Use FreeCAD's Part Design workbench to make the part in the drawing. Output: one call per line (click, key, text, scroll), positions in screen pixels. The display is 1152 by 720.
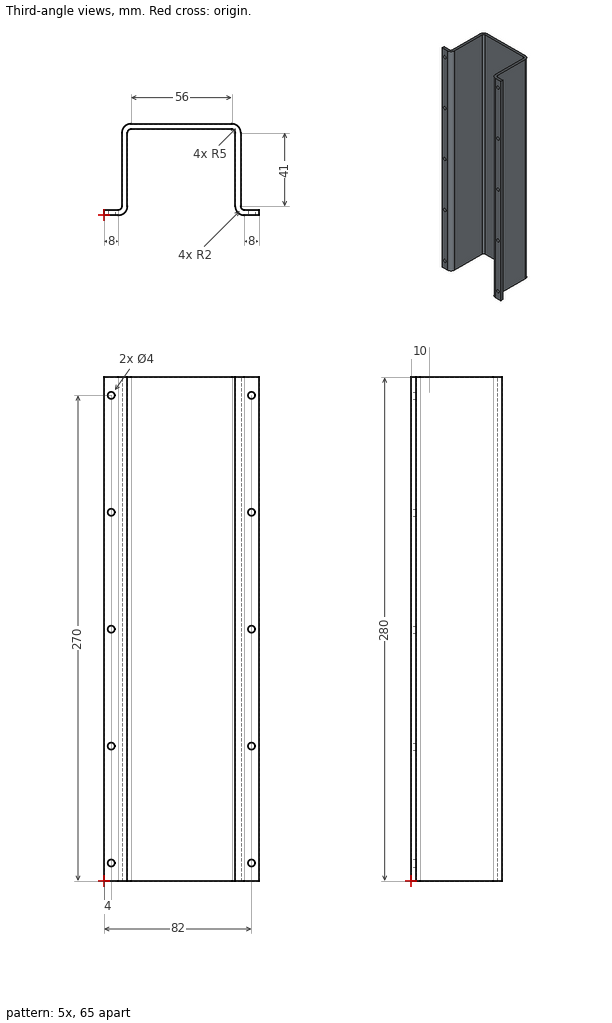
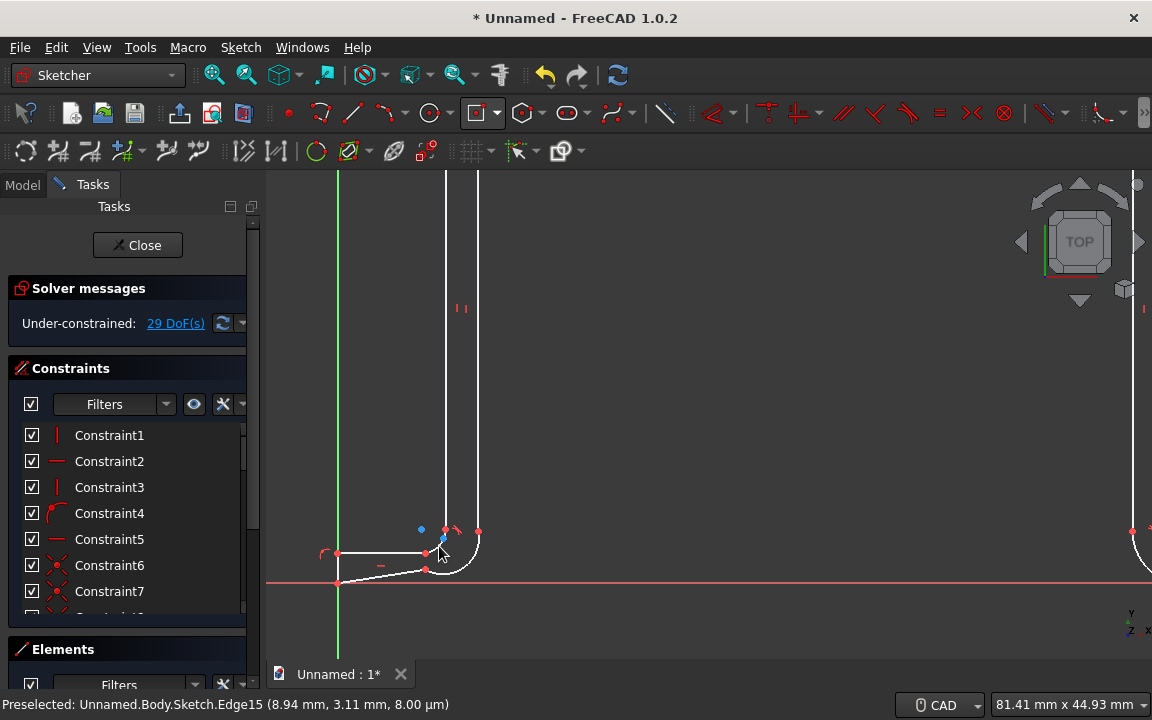
click(399, 553)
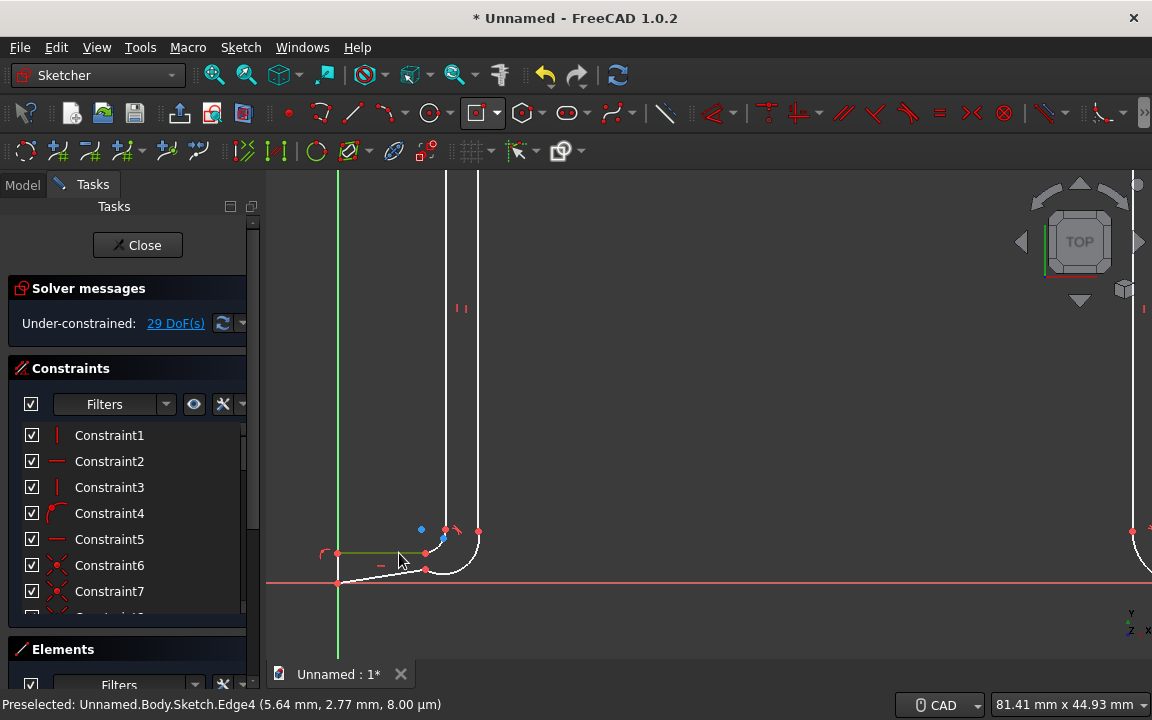
scroll(435, 550, up, 2)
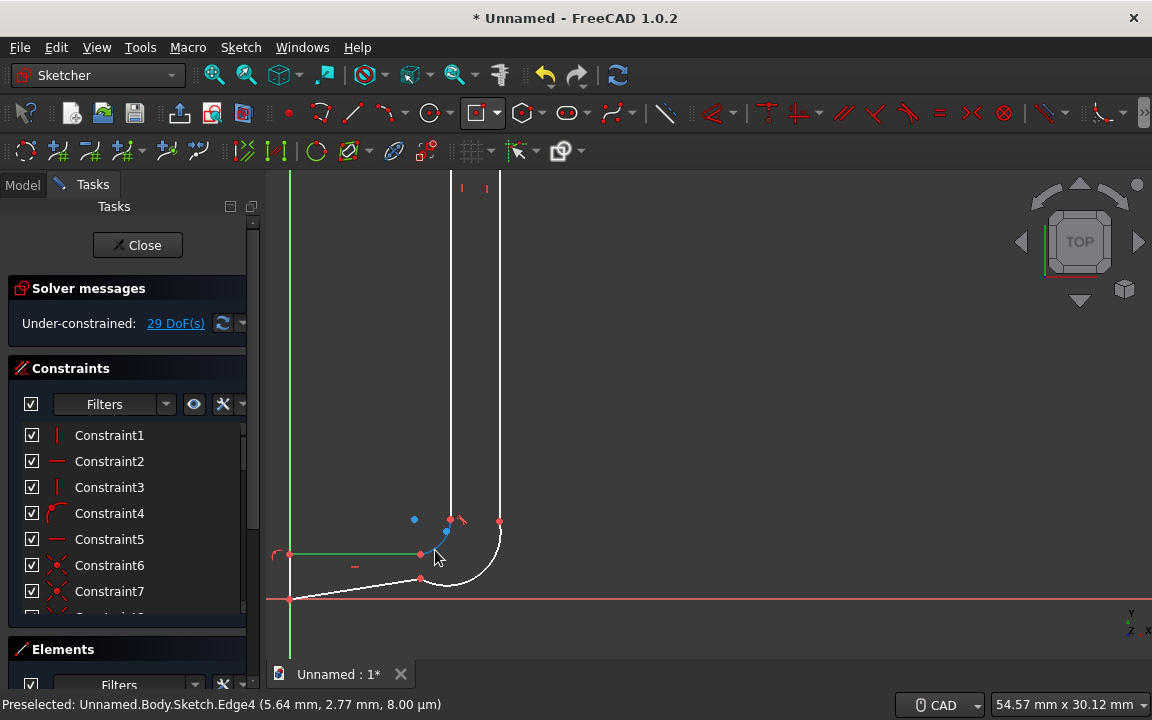
click(435, 549)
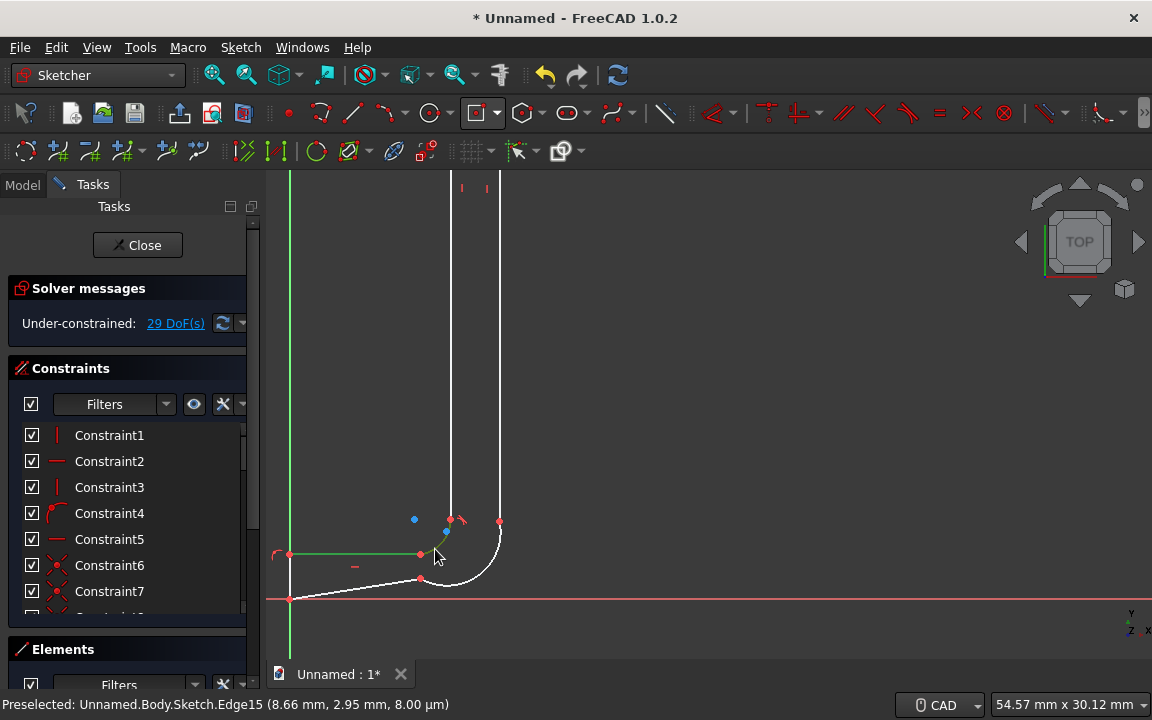
key(t)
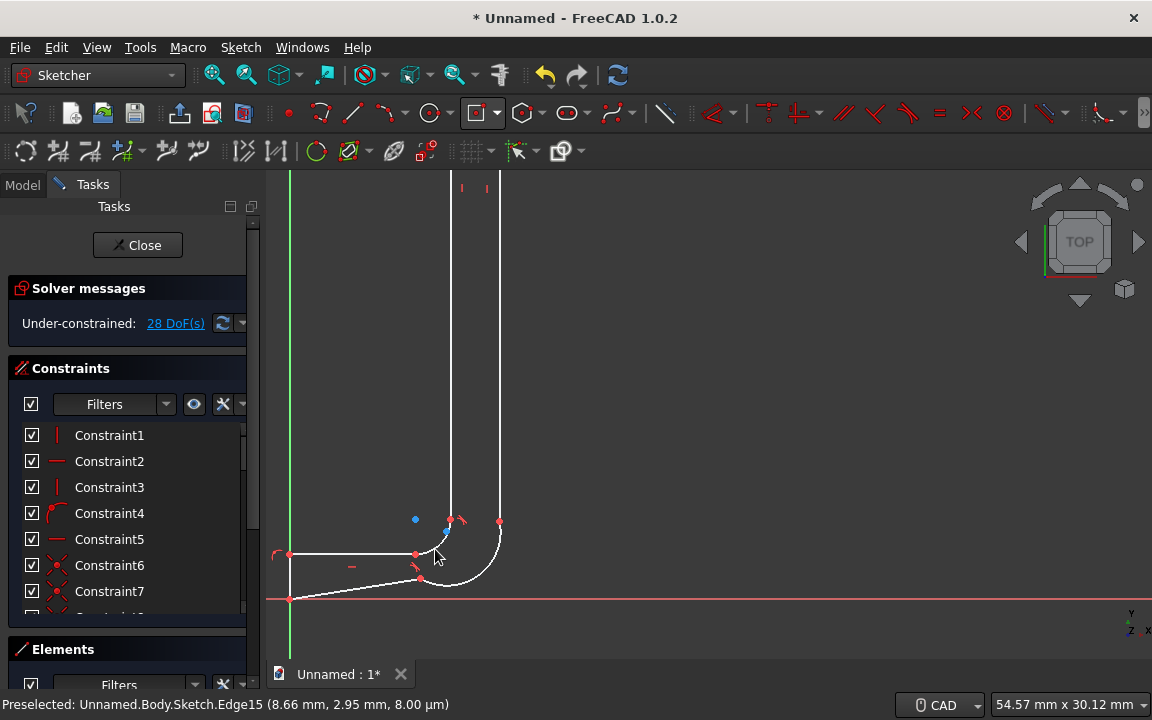
click(381, 585)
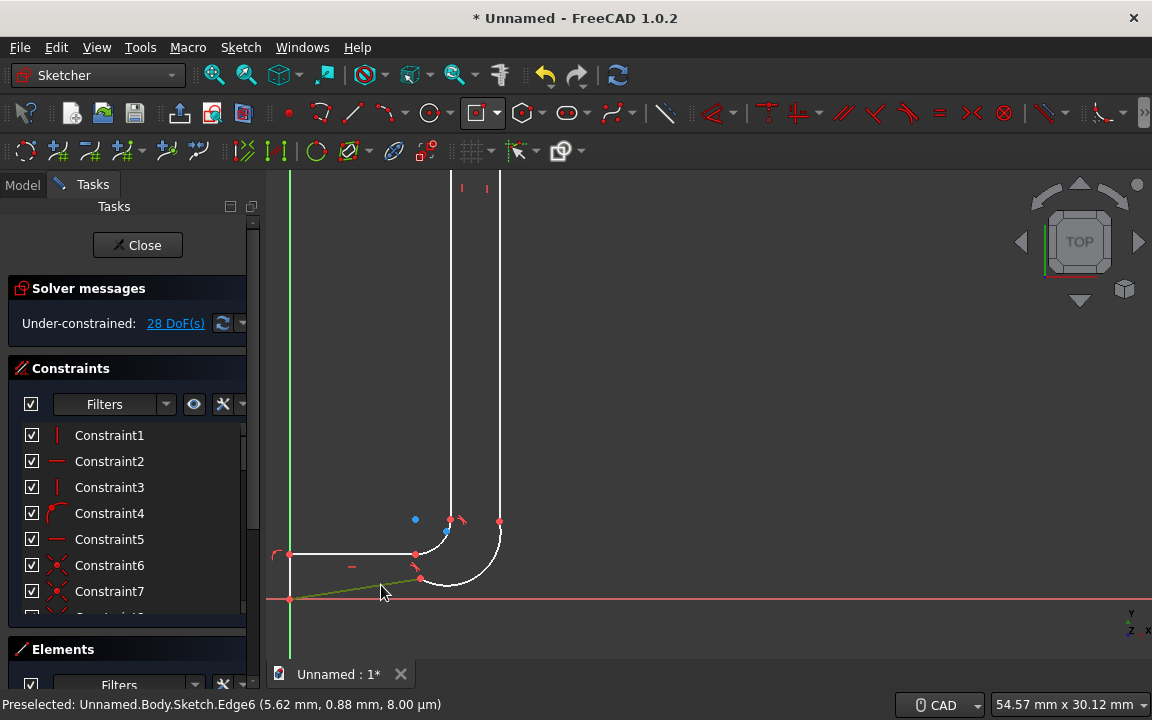
click(456, 585)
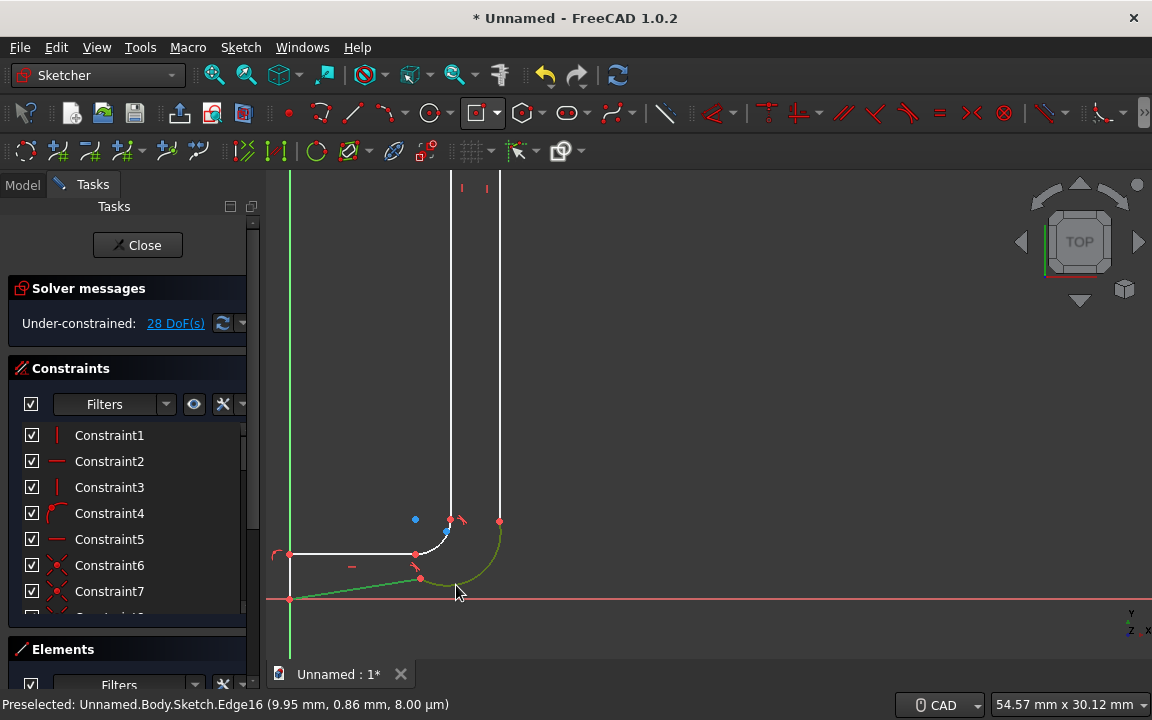
key(t)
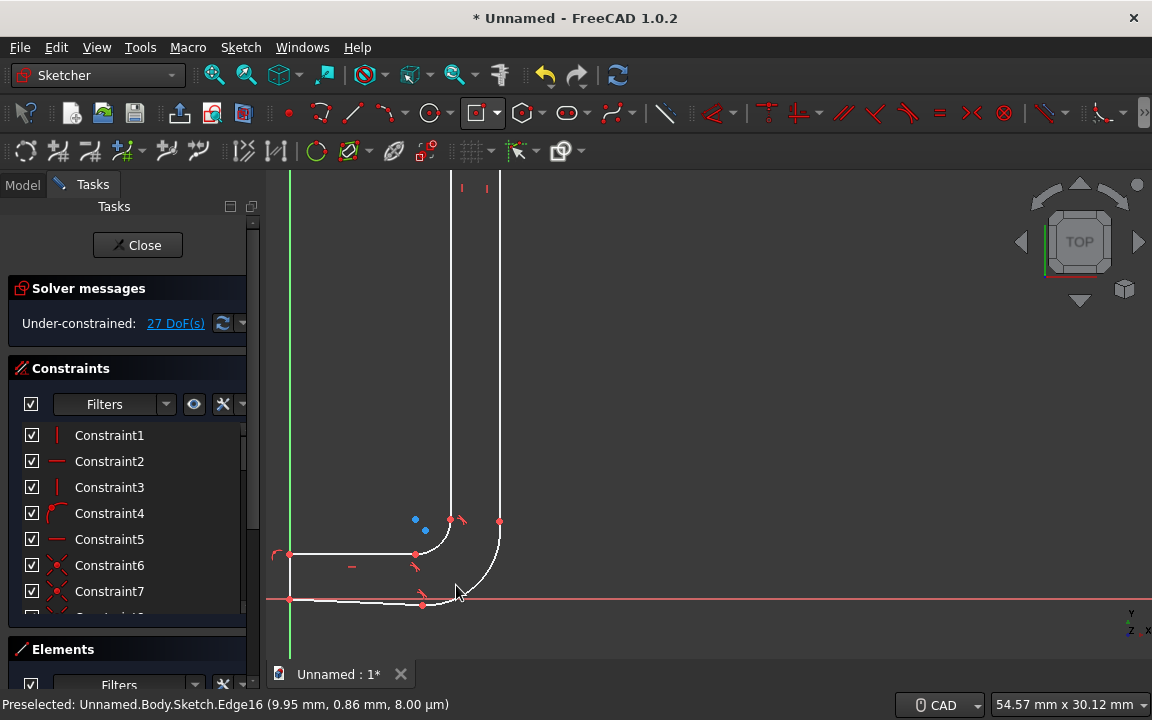
click(500, 322)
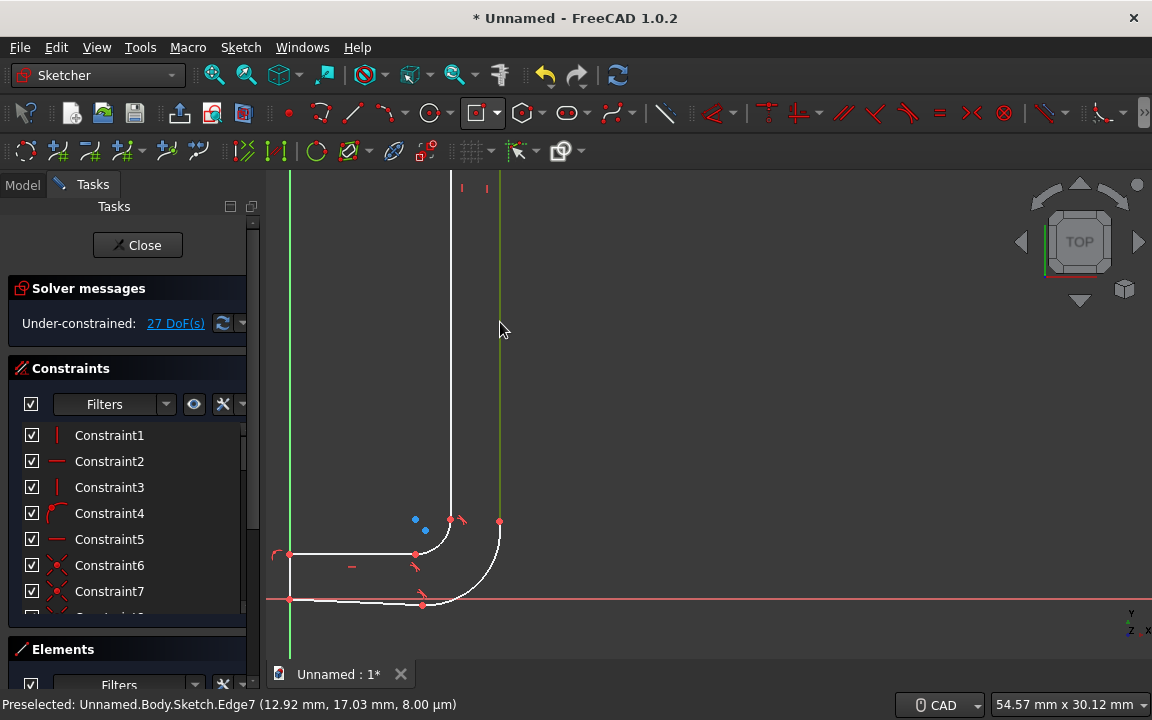
click(460, 597)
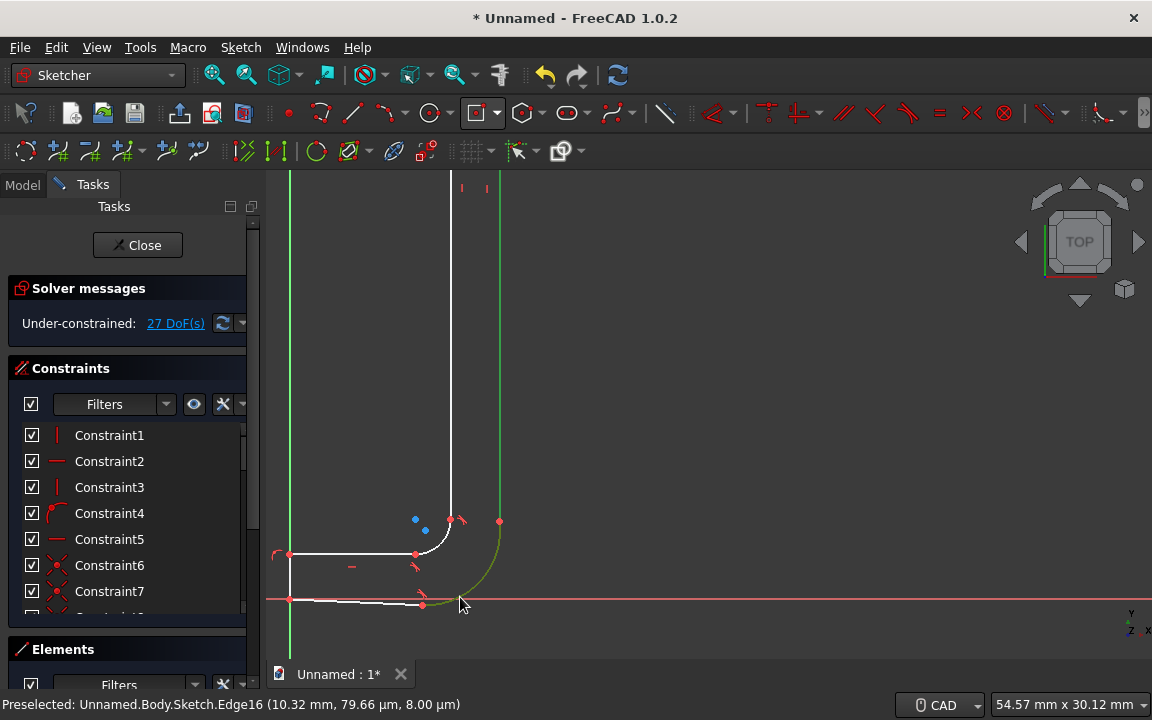
click(908, 114)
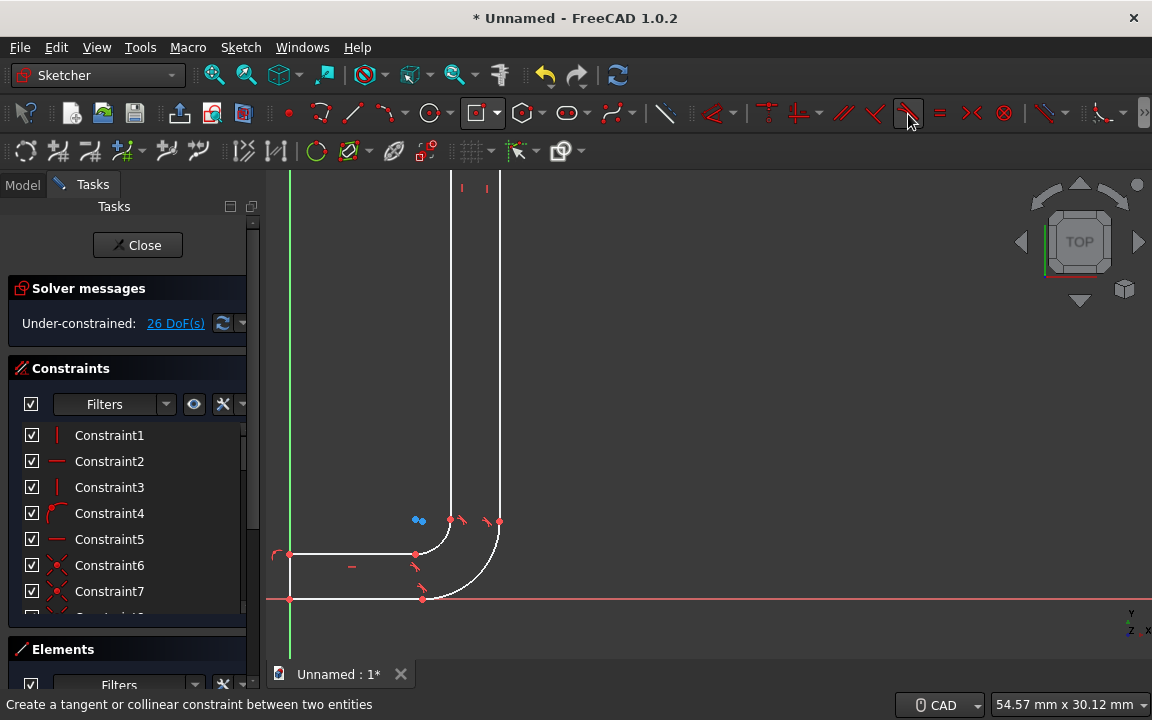
click(500, 322)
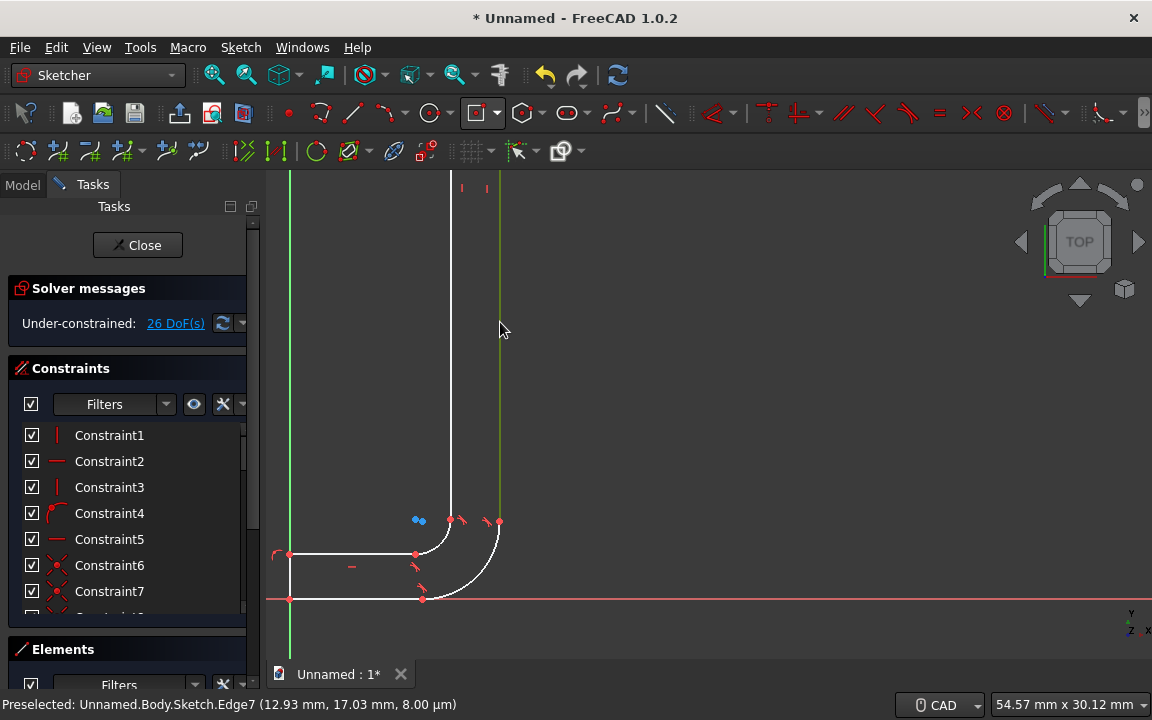
scroll(438, 548, down, 5)